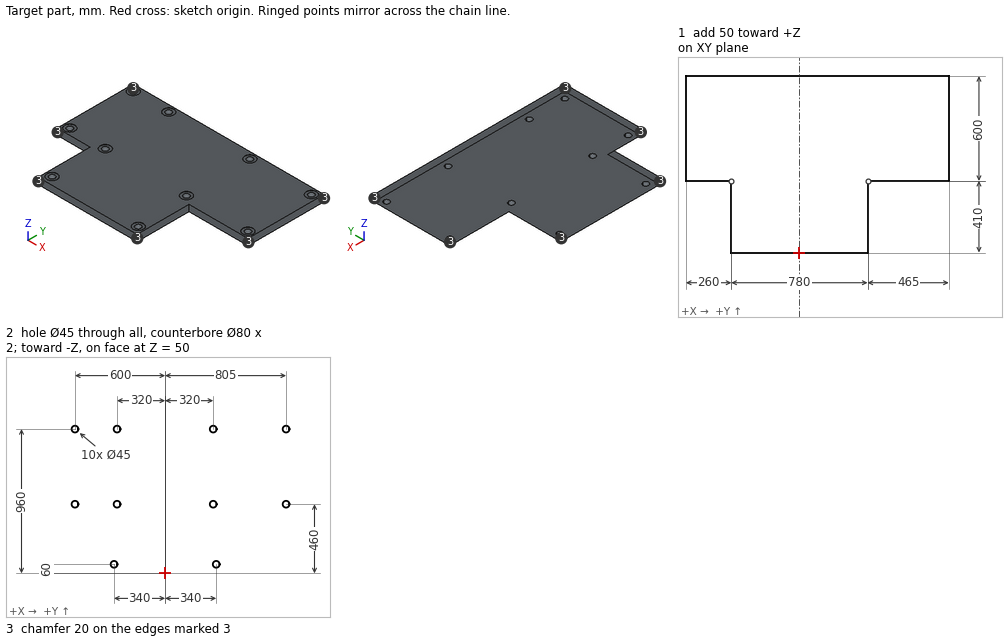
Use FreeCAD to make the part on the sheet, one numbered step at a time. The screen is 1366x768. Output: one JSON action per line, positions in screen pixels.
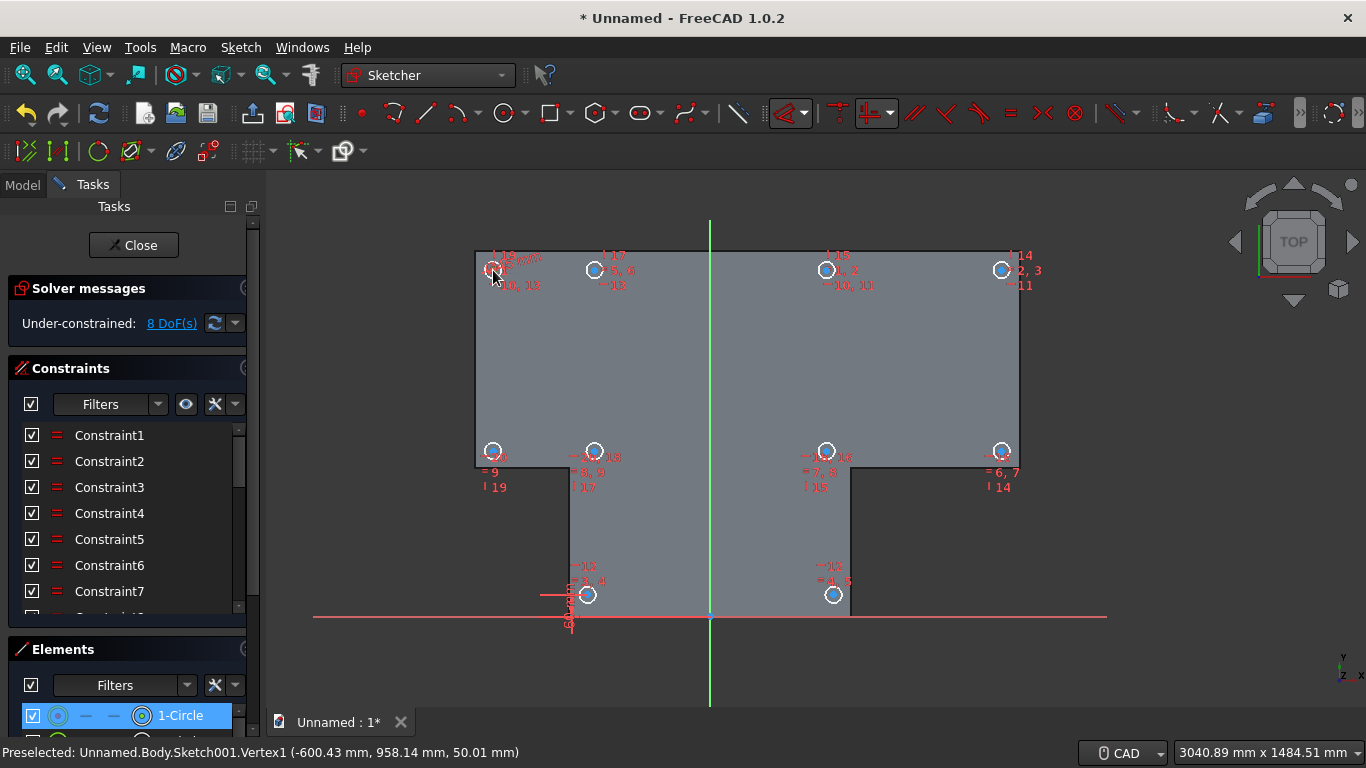
{"action": "key", "text": "l"}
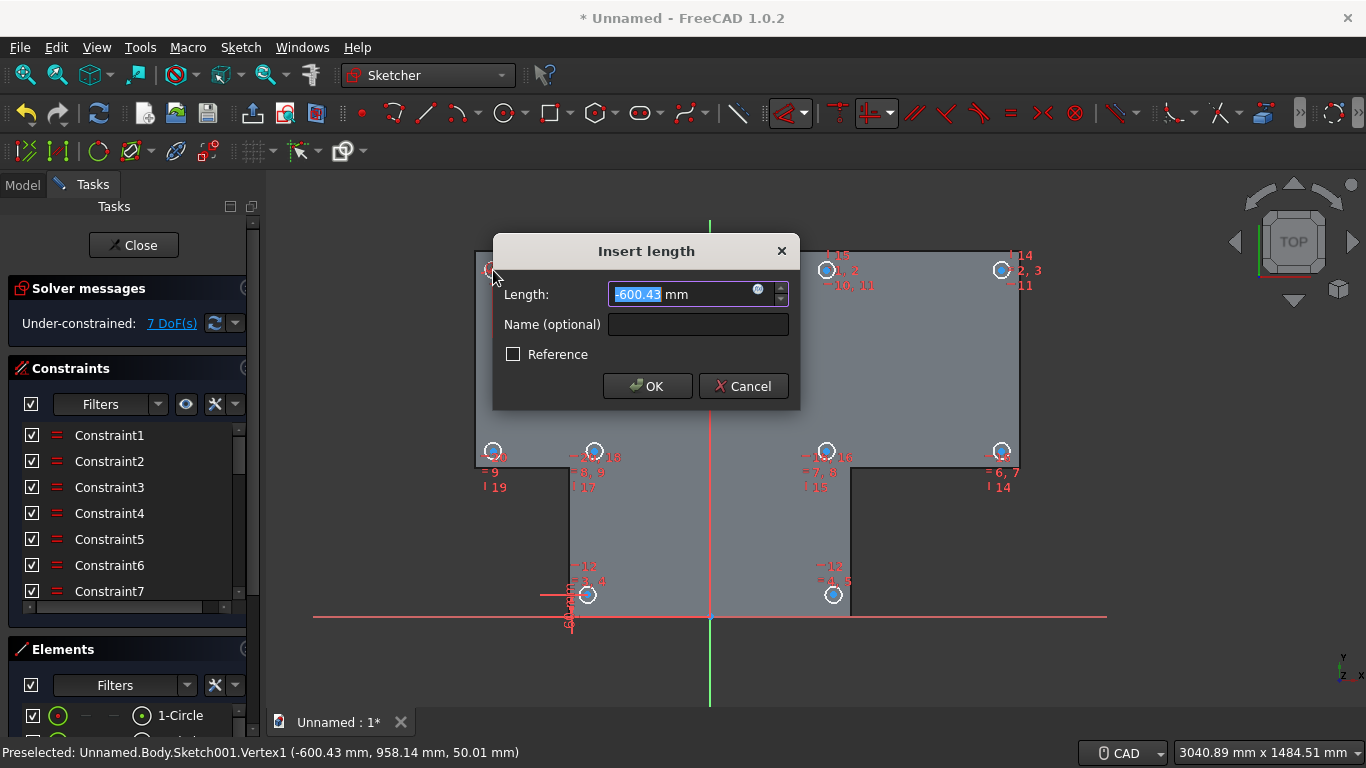
{"action": "type", "text": "-600"}
{"action": "key", "text": "Return"}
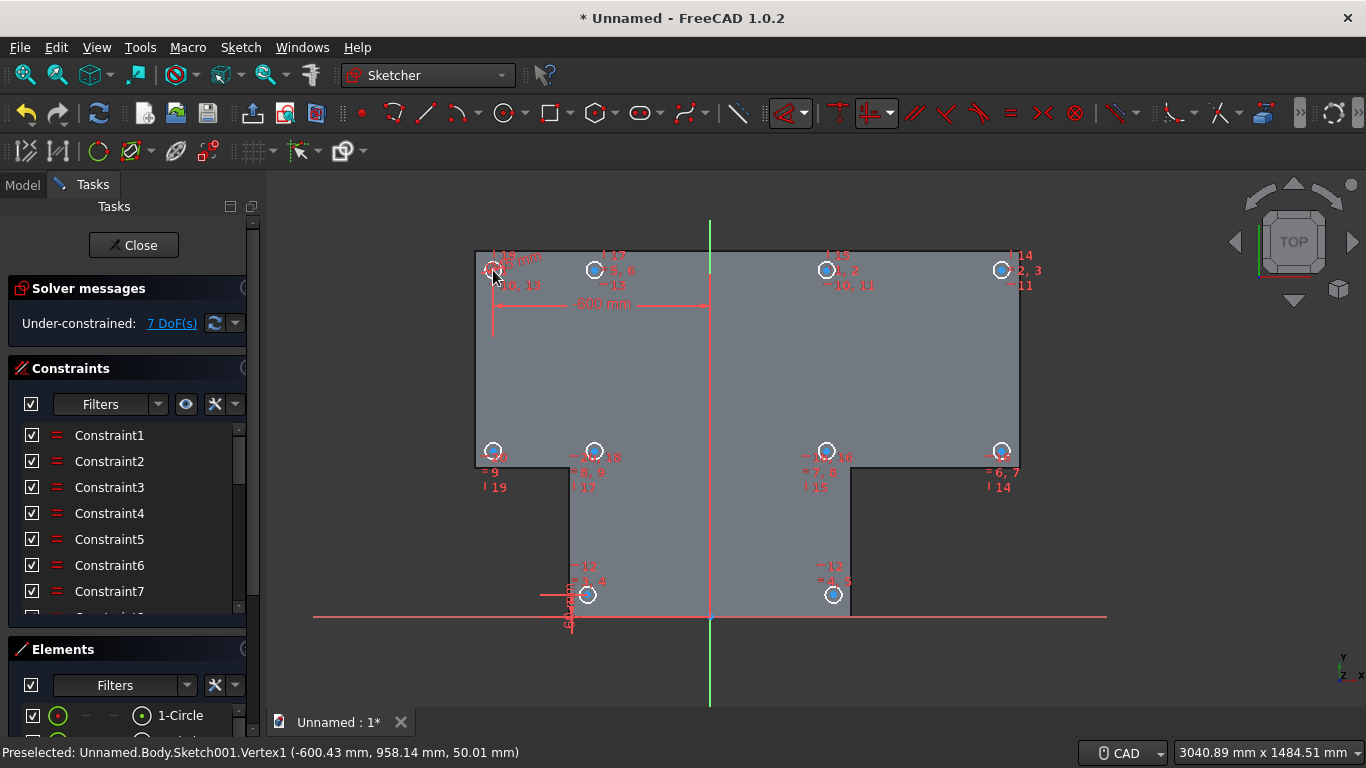
{"action": "left_click", "coordinate": [493, 270]}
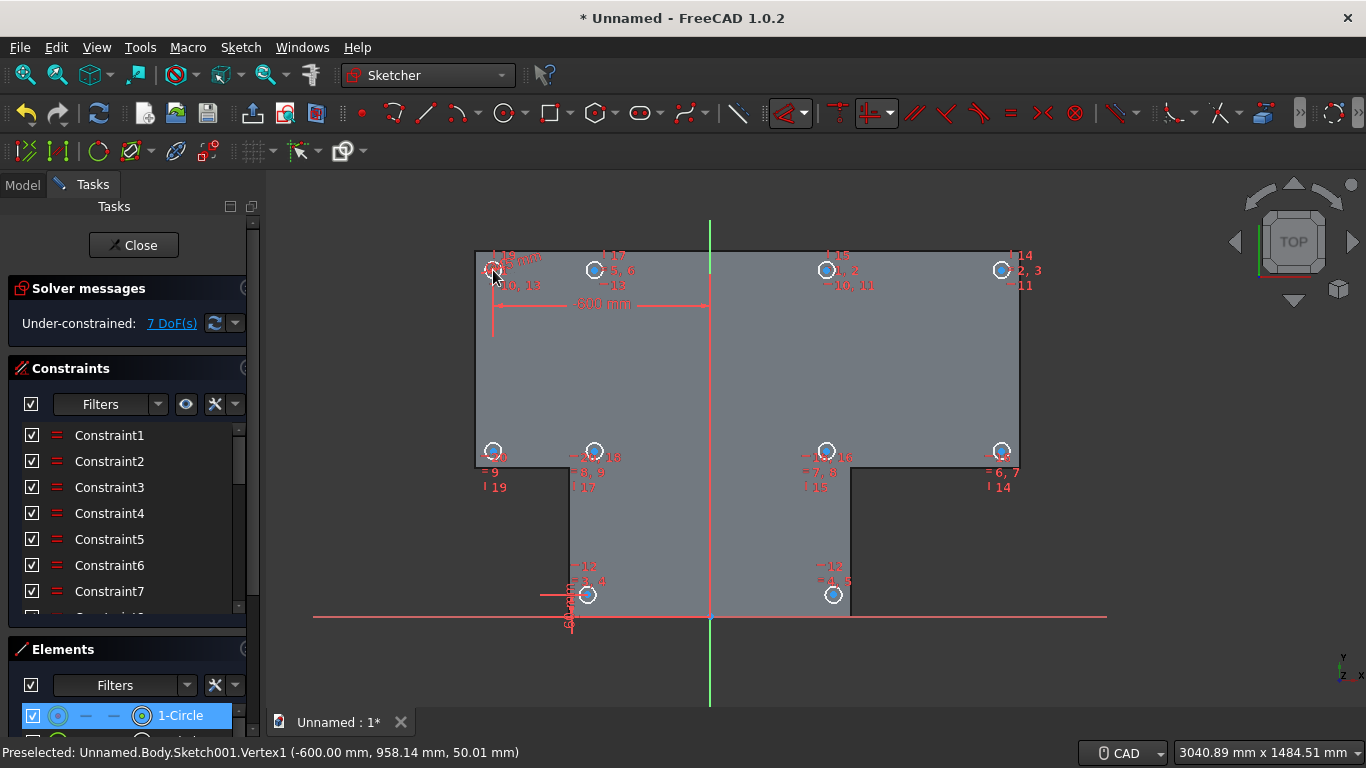
{"action": "key", "text": "i"}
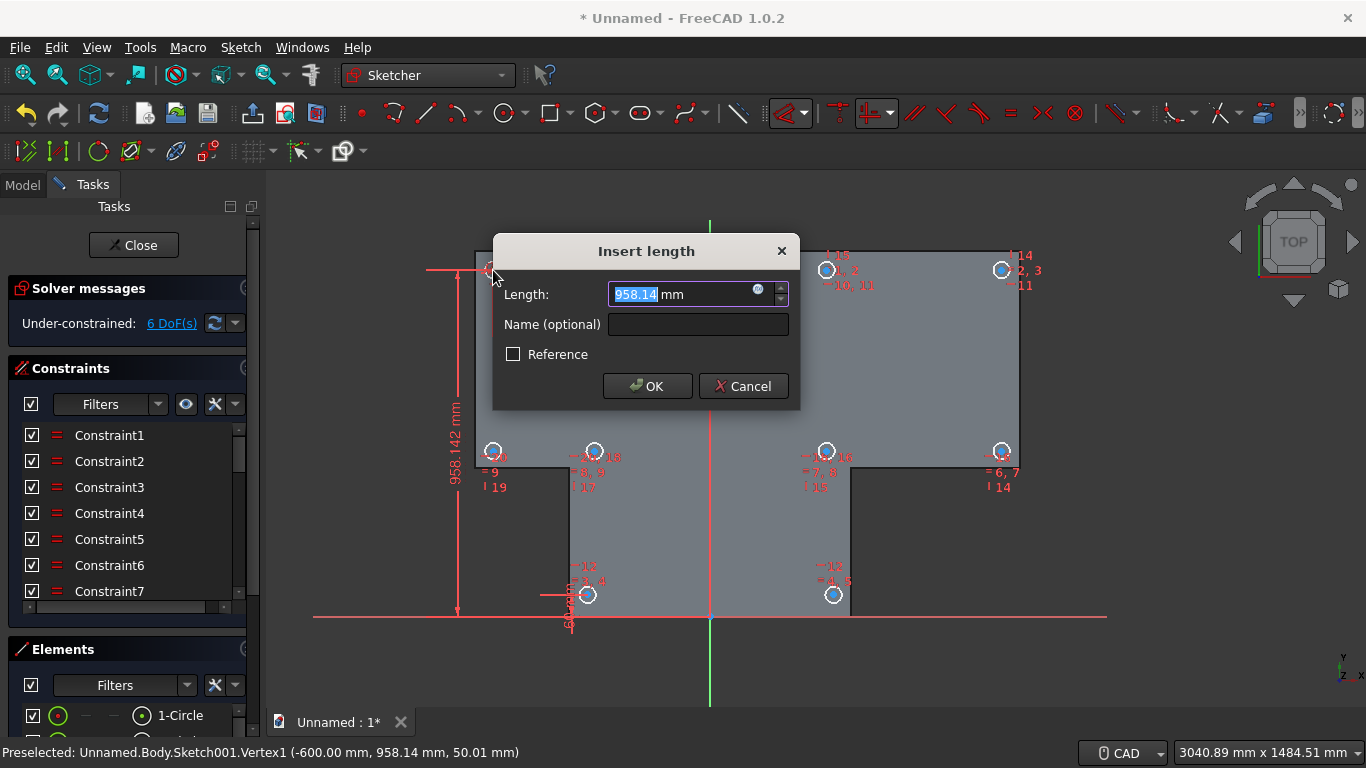
{"action": "type", "text": "960"}
{"action": "key", "text": "Return"}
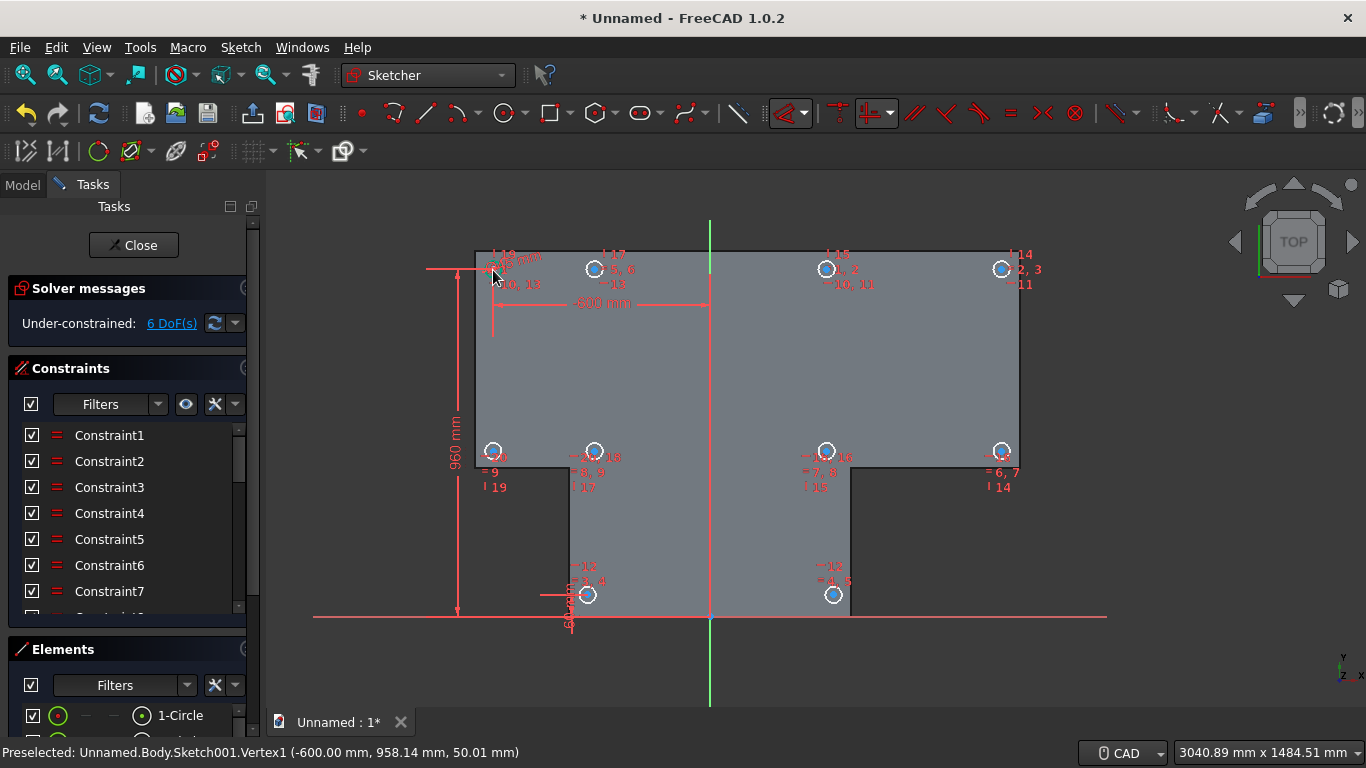
{"action": "left_click", "coordinate": [827, 269]}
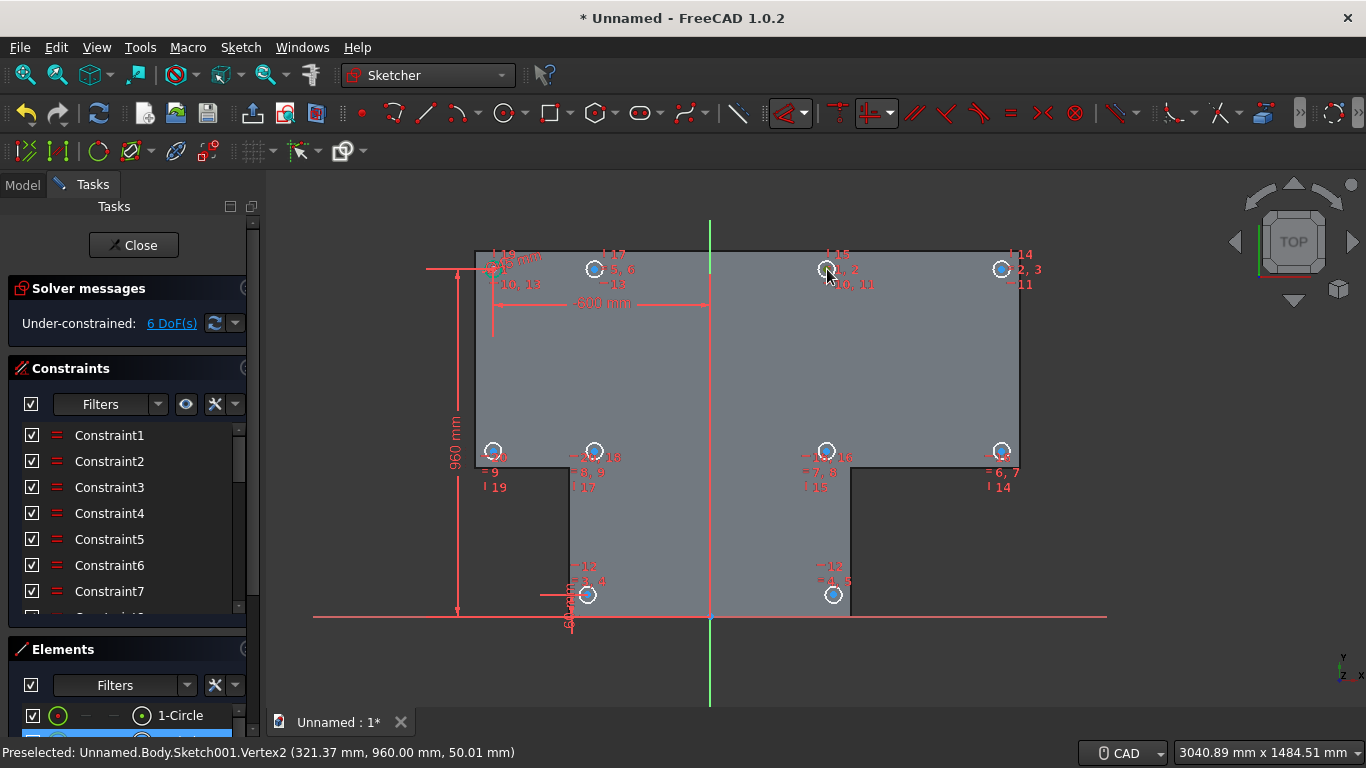
{"action": "left_click", "coordinate": [806, 114]}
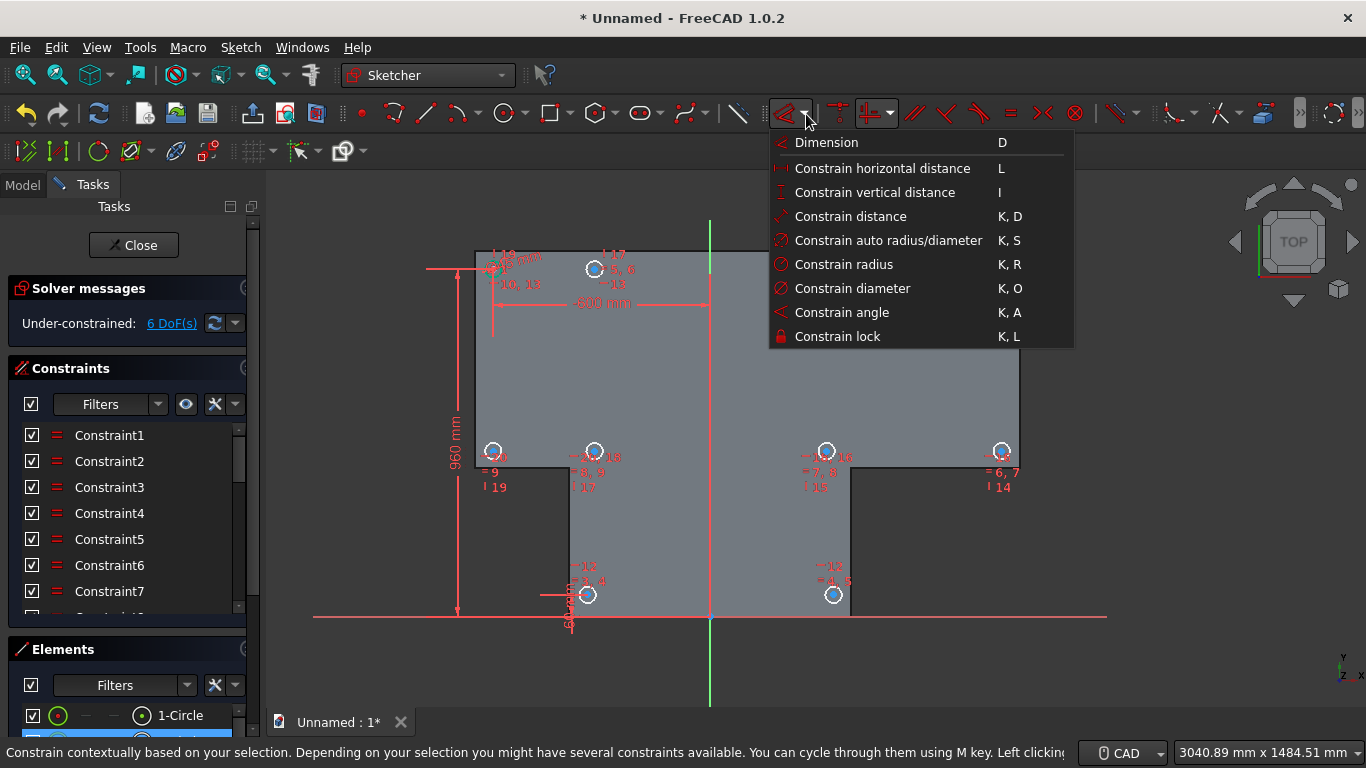
{"action": "left_click", "coordinate": [922, 168]}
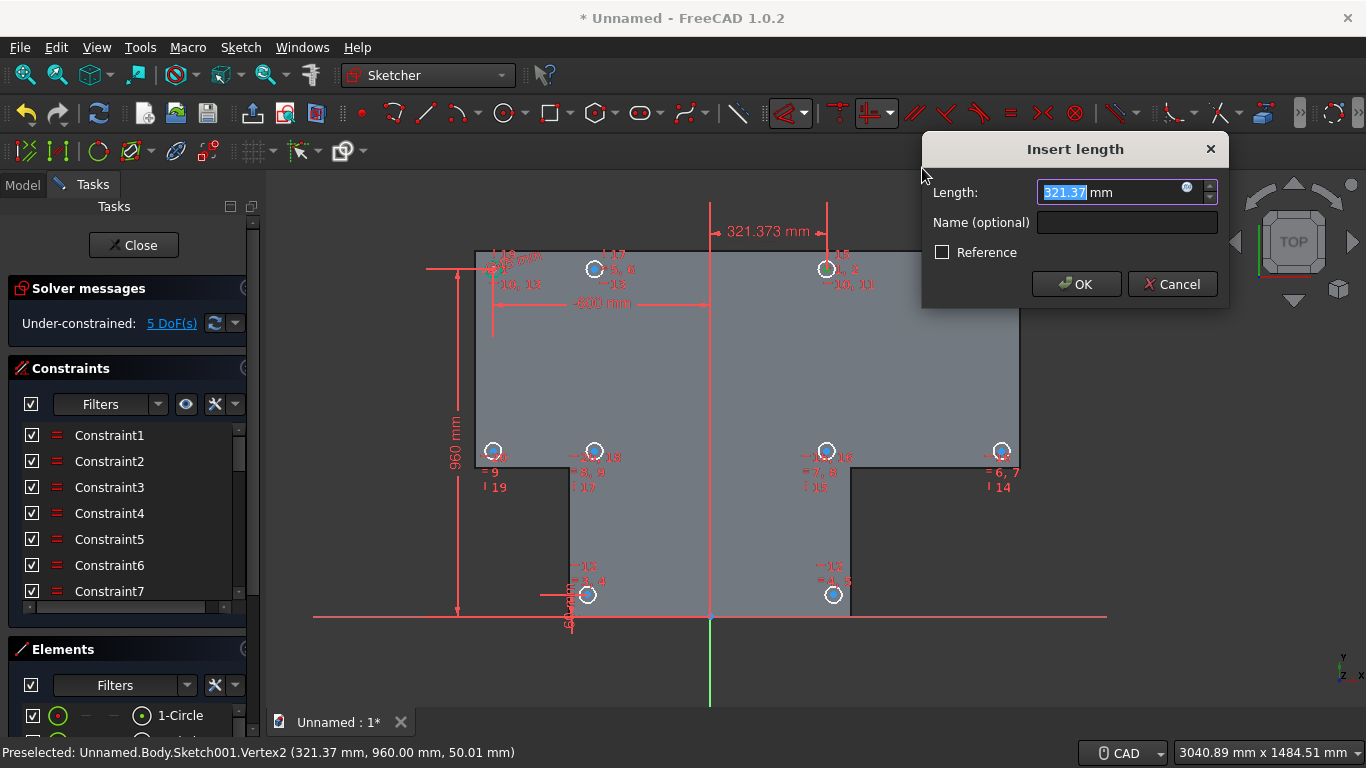
{"action": "type", "text": "320"}
{"action": "key", "text": "Return"}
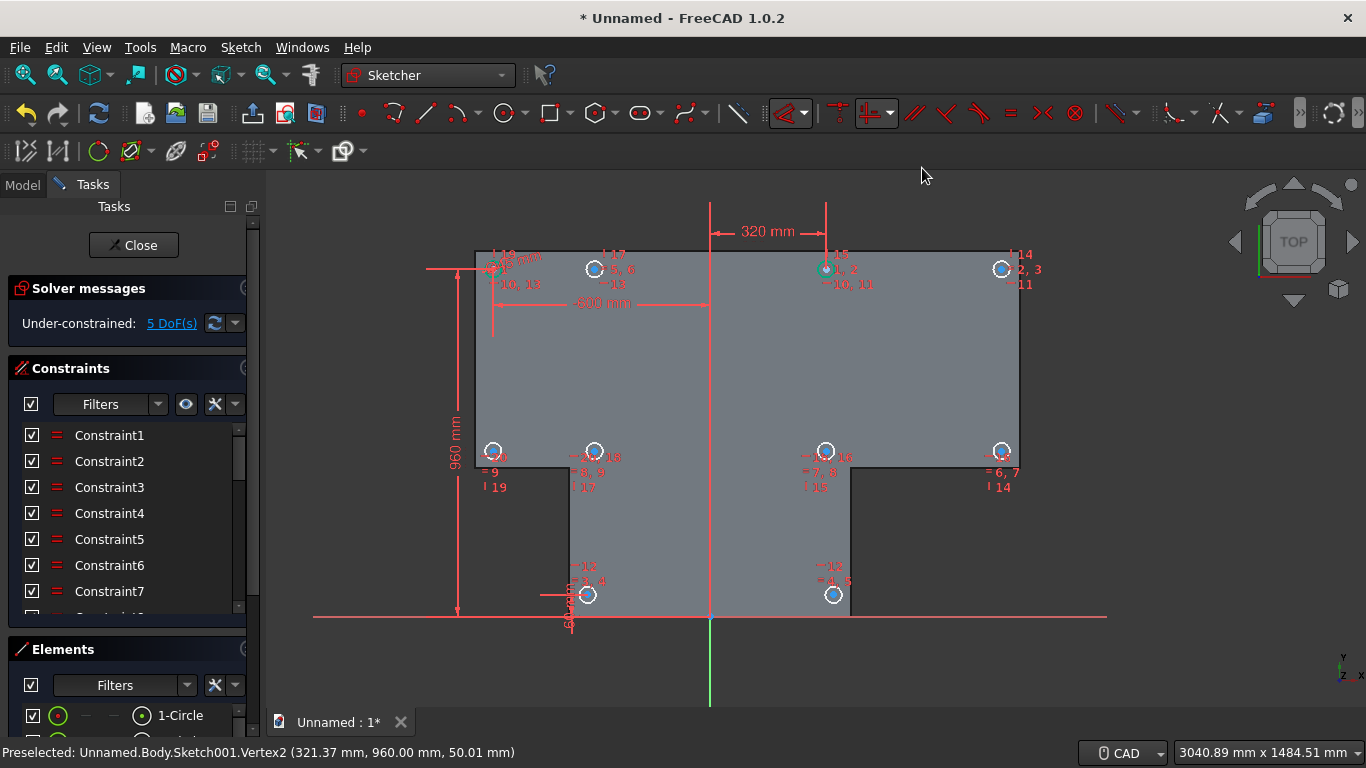
{"action": "left_click", "coordinate": [1002, 269]}